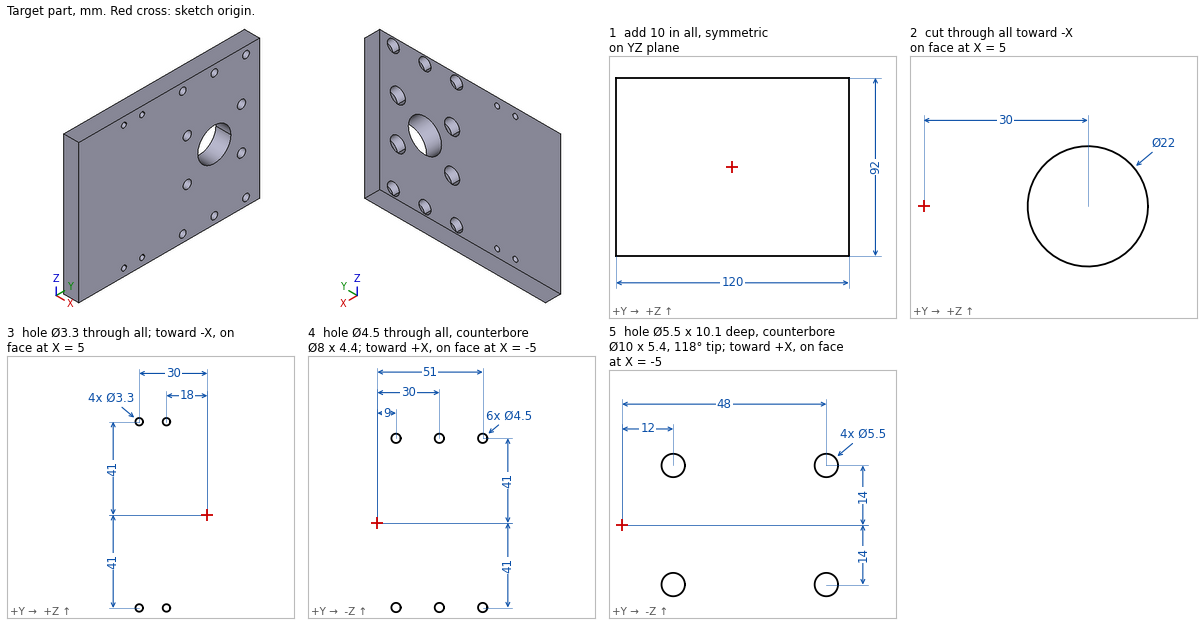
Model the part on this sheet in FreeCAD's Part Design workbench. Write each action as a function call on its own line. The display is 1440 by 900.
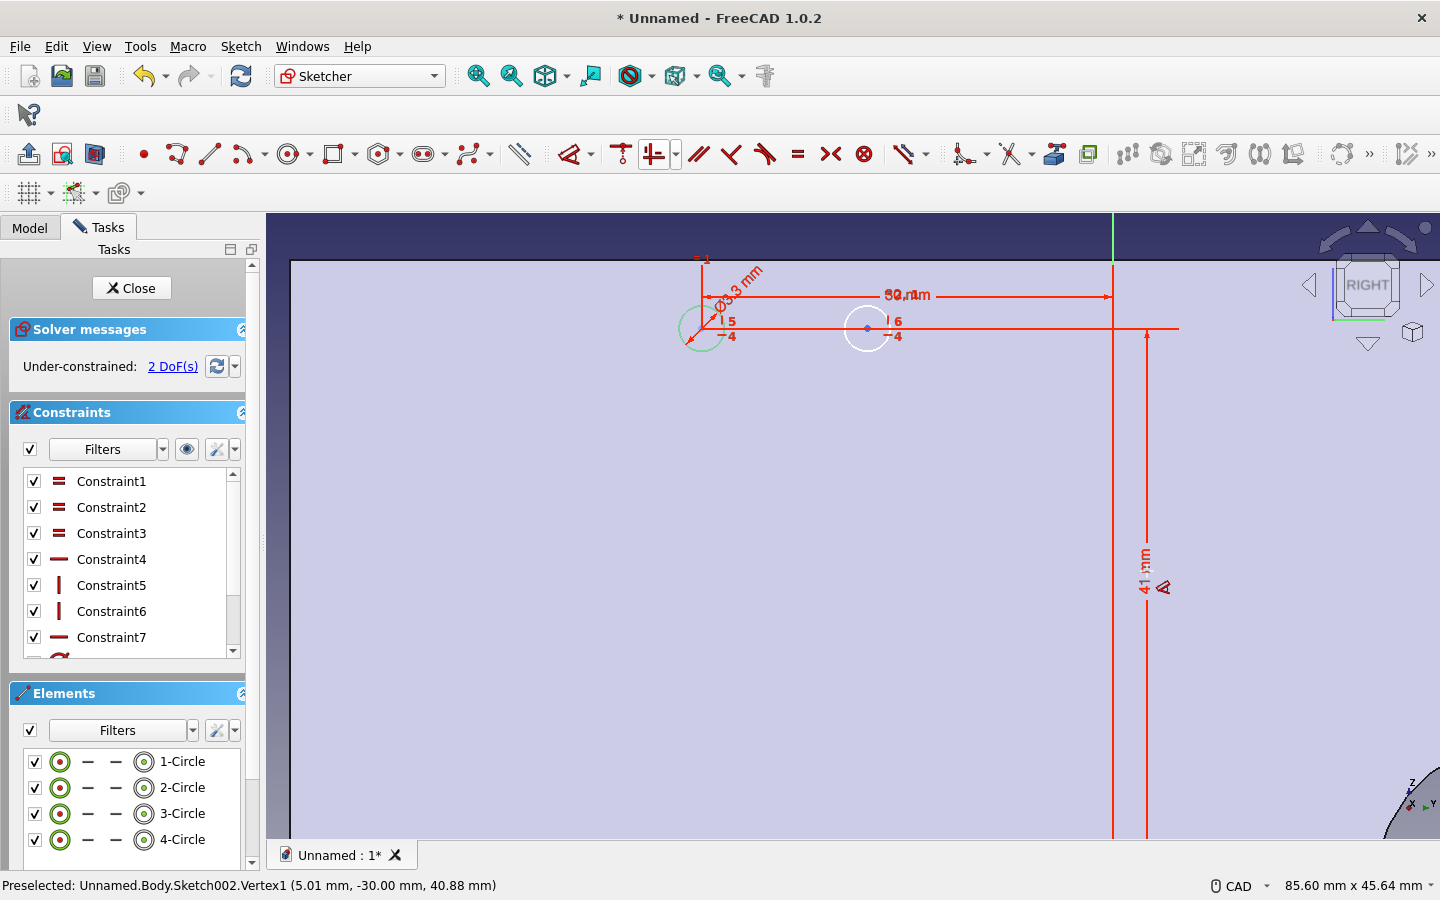
click(867, 329)
click(990, 295)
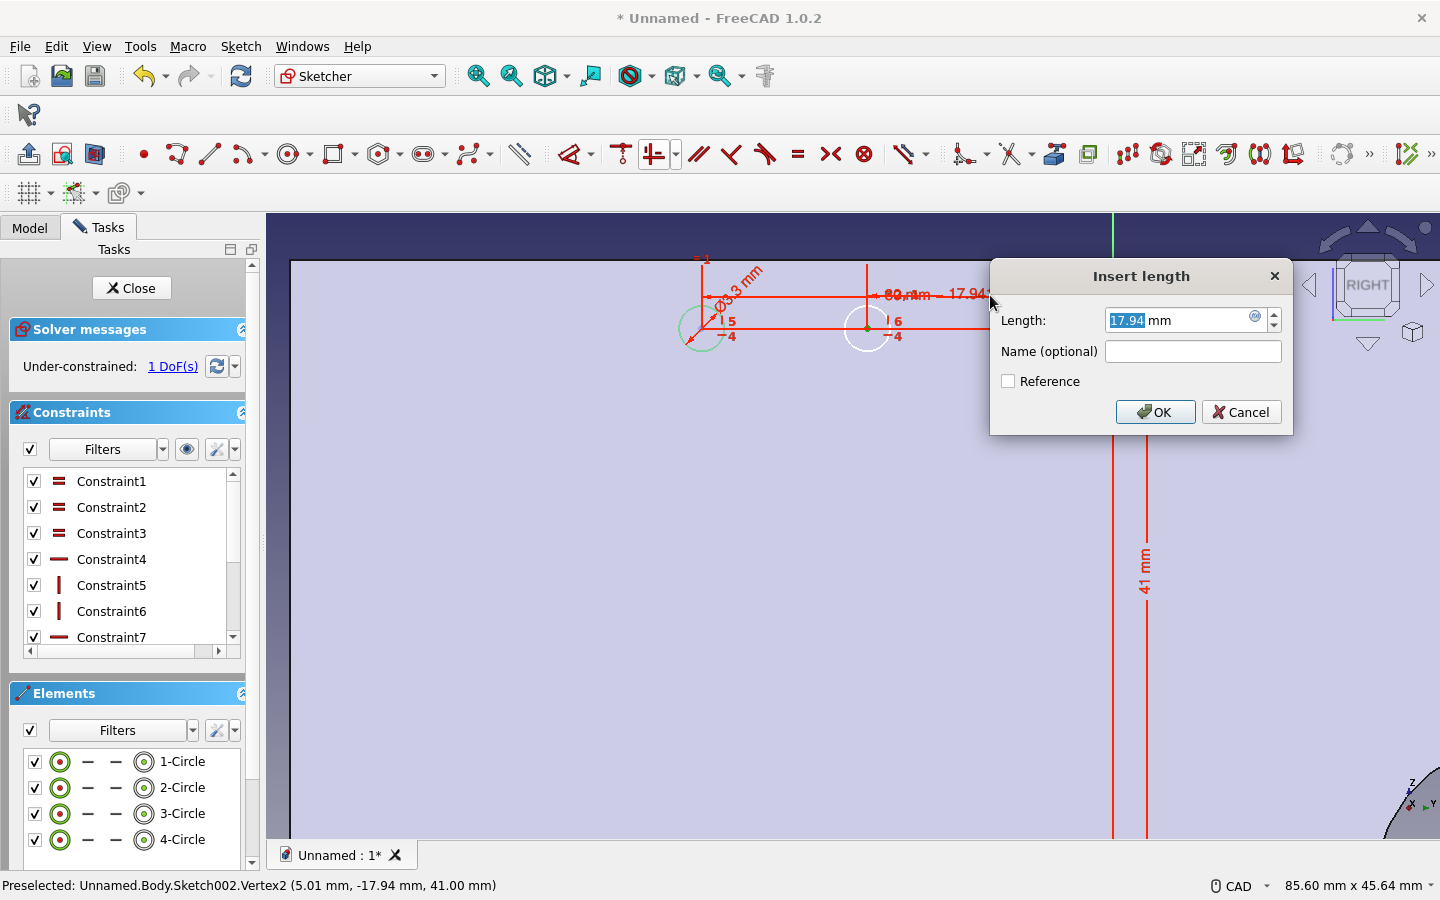
text(18)
key(Return)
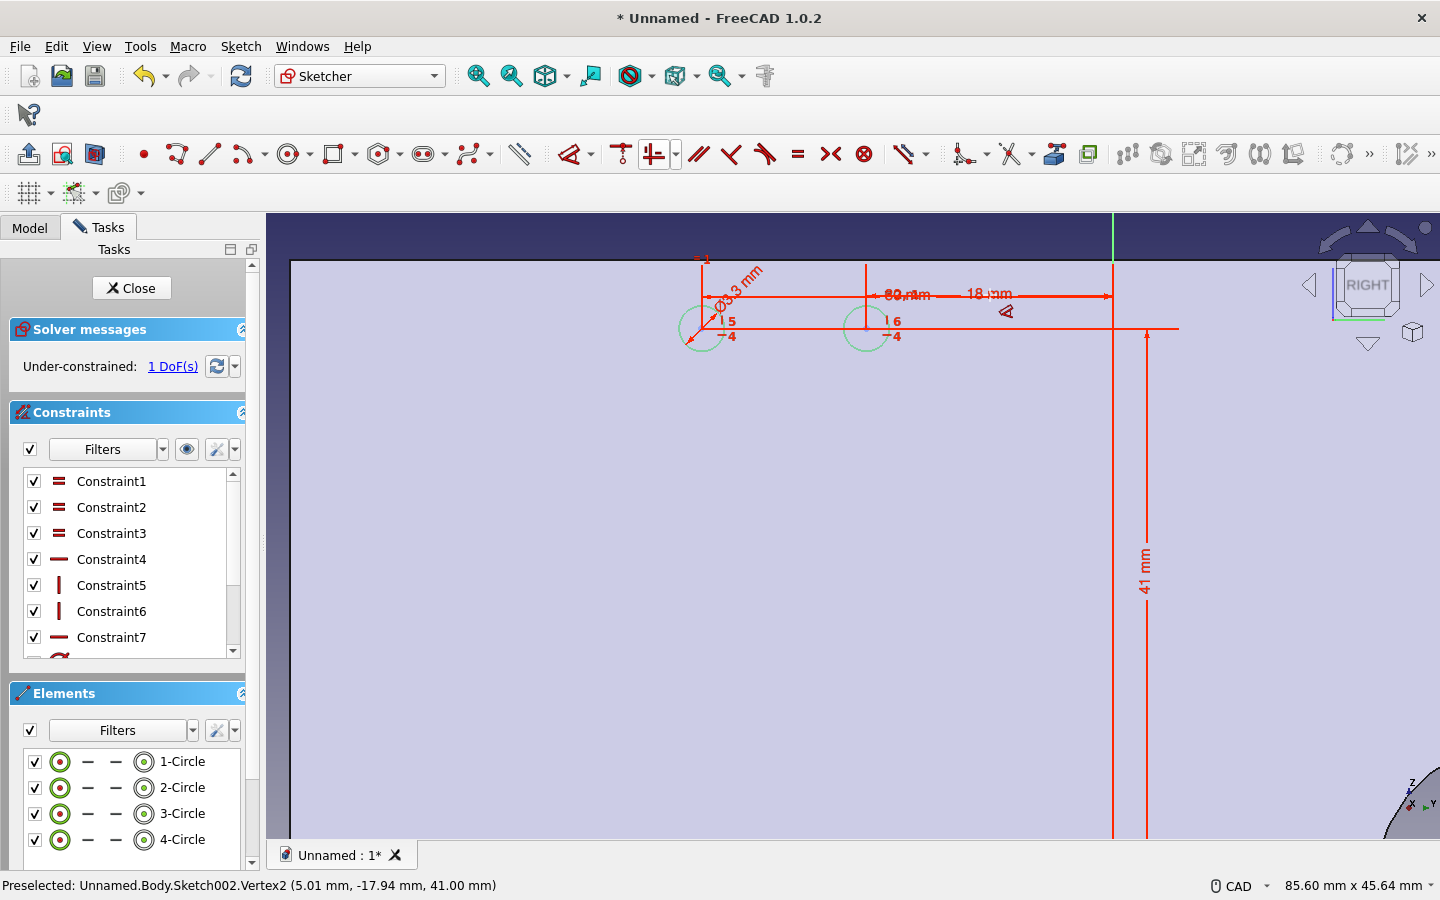
scroll(719, 314, down, 5)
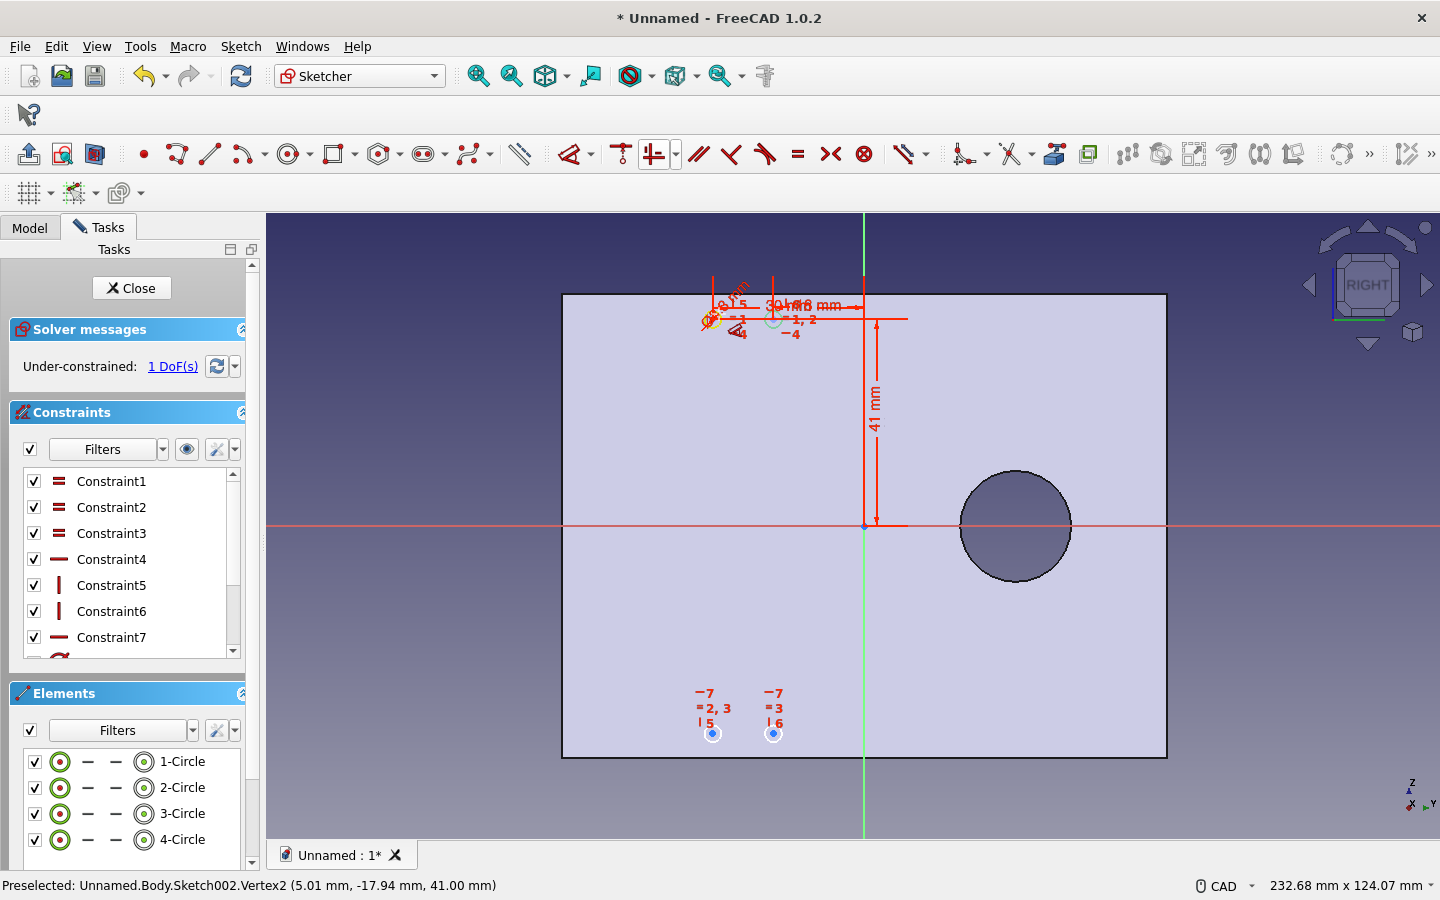
click(713, 734)
click(898, 630)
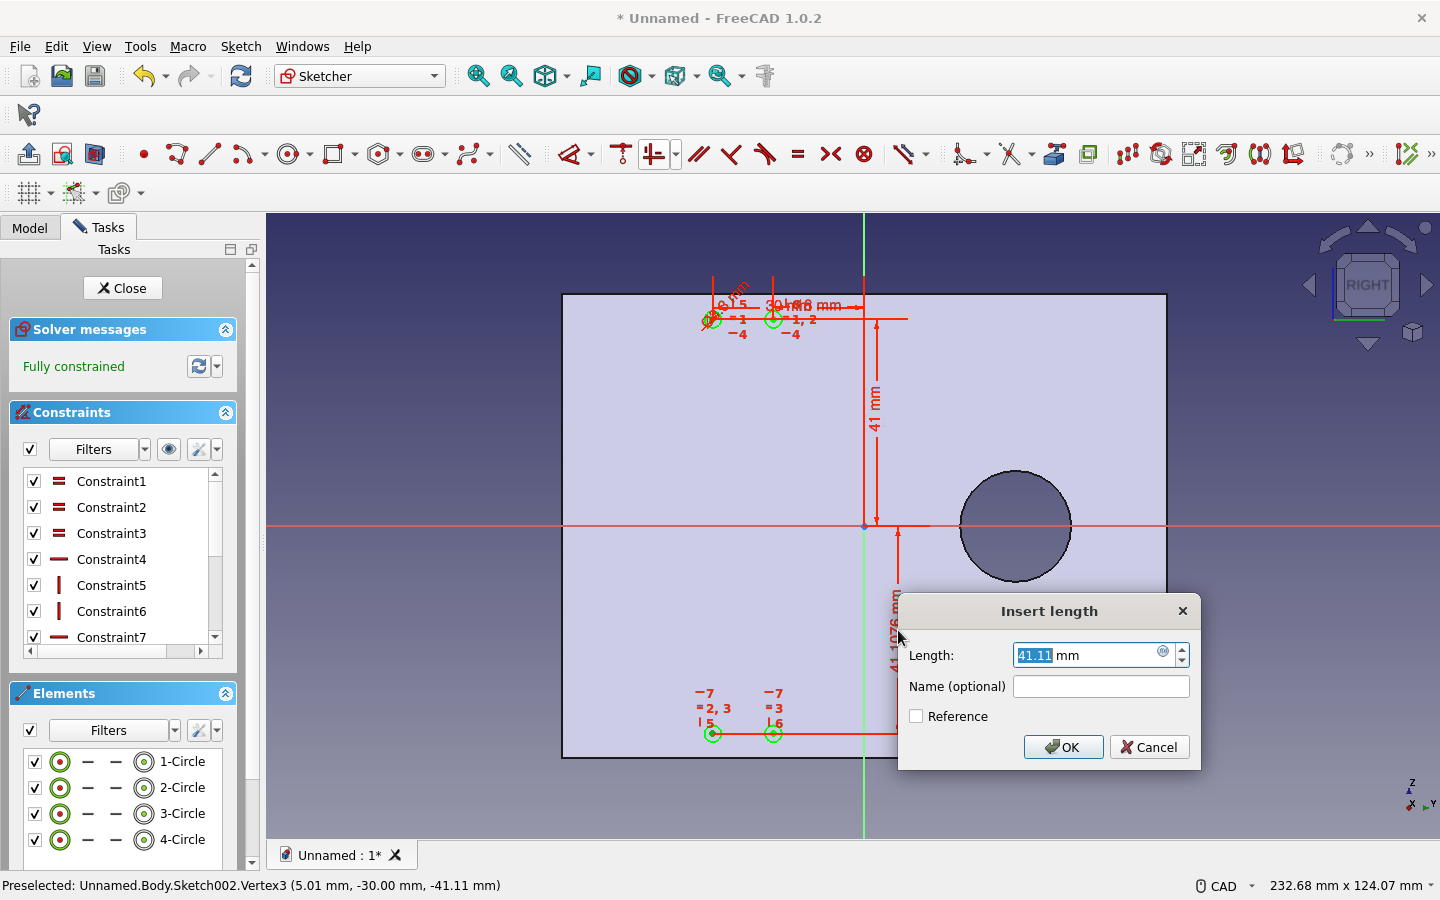
text(41)
key(Return)
key(Escape)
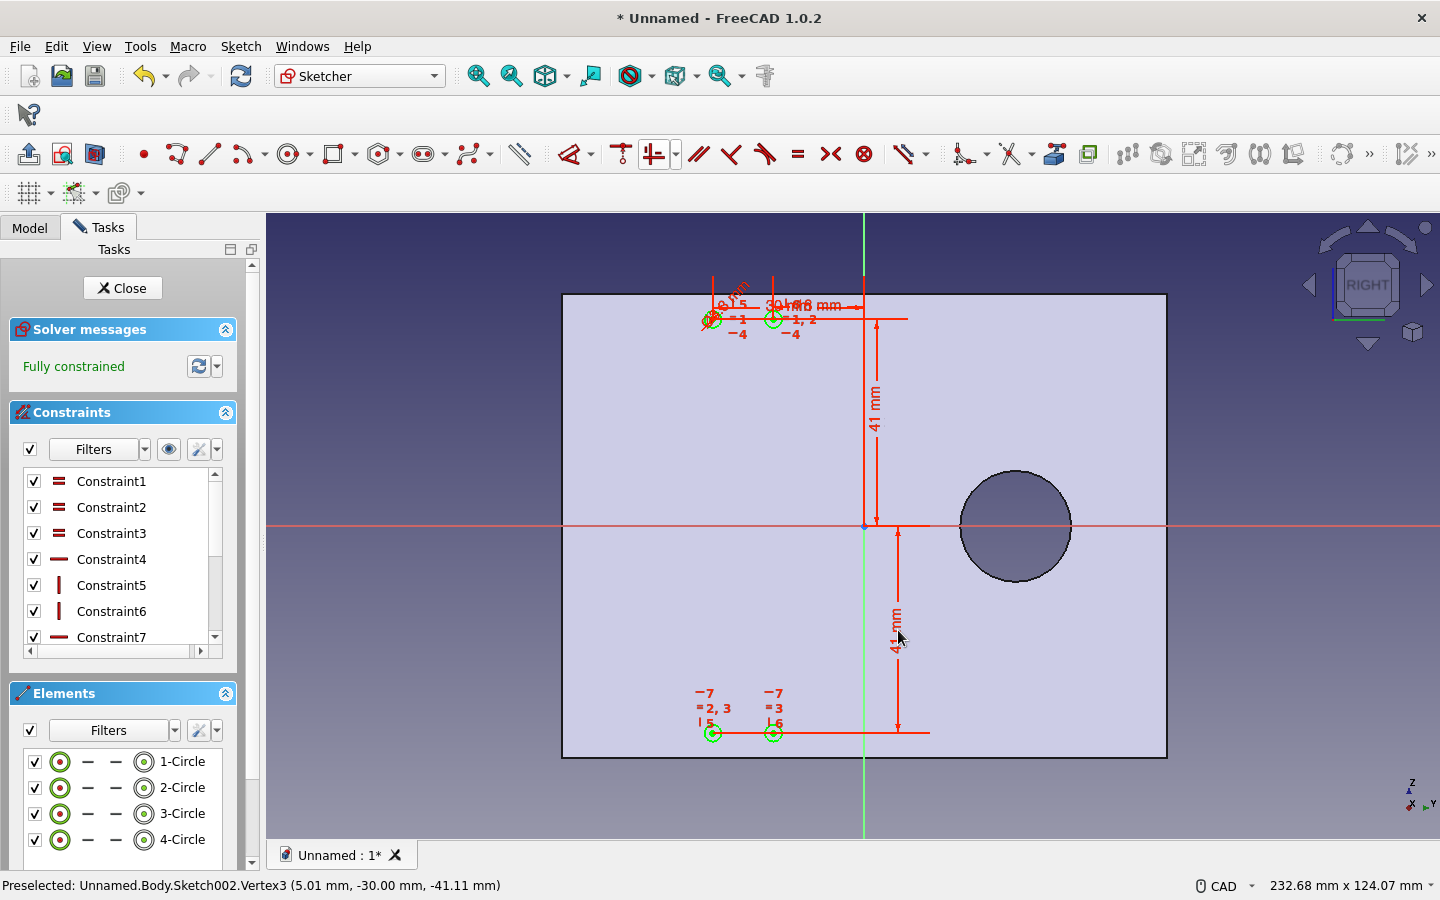
click(123, 288)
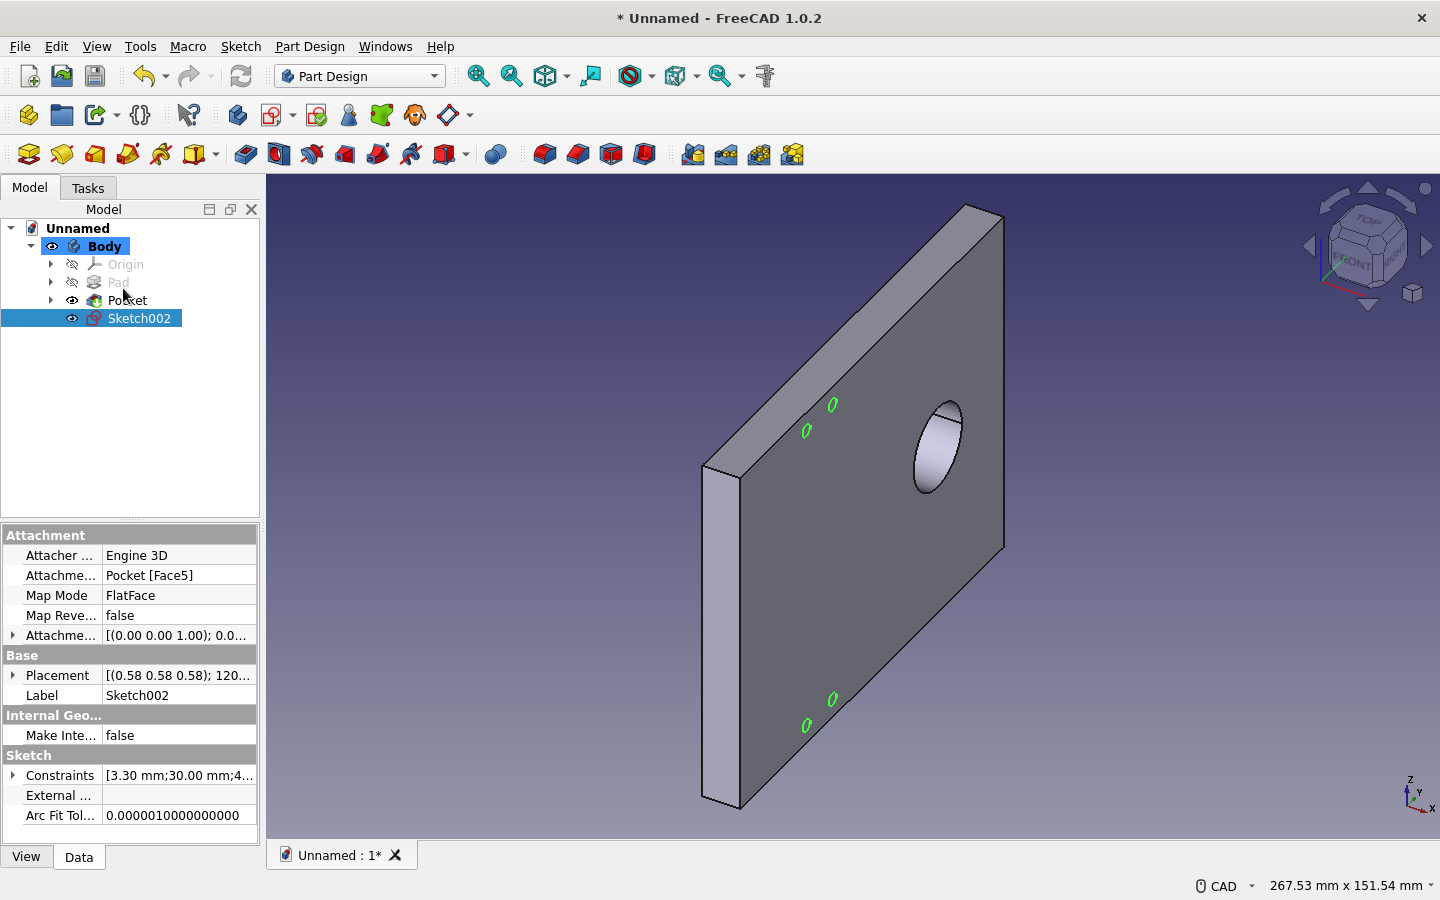
click(279, 154)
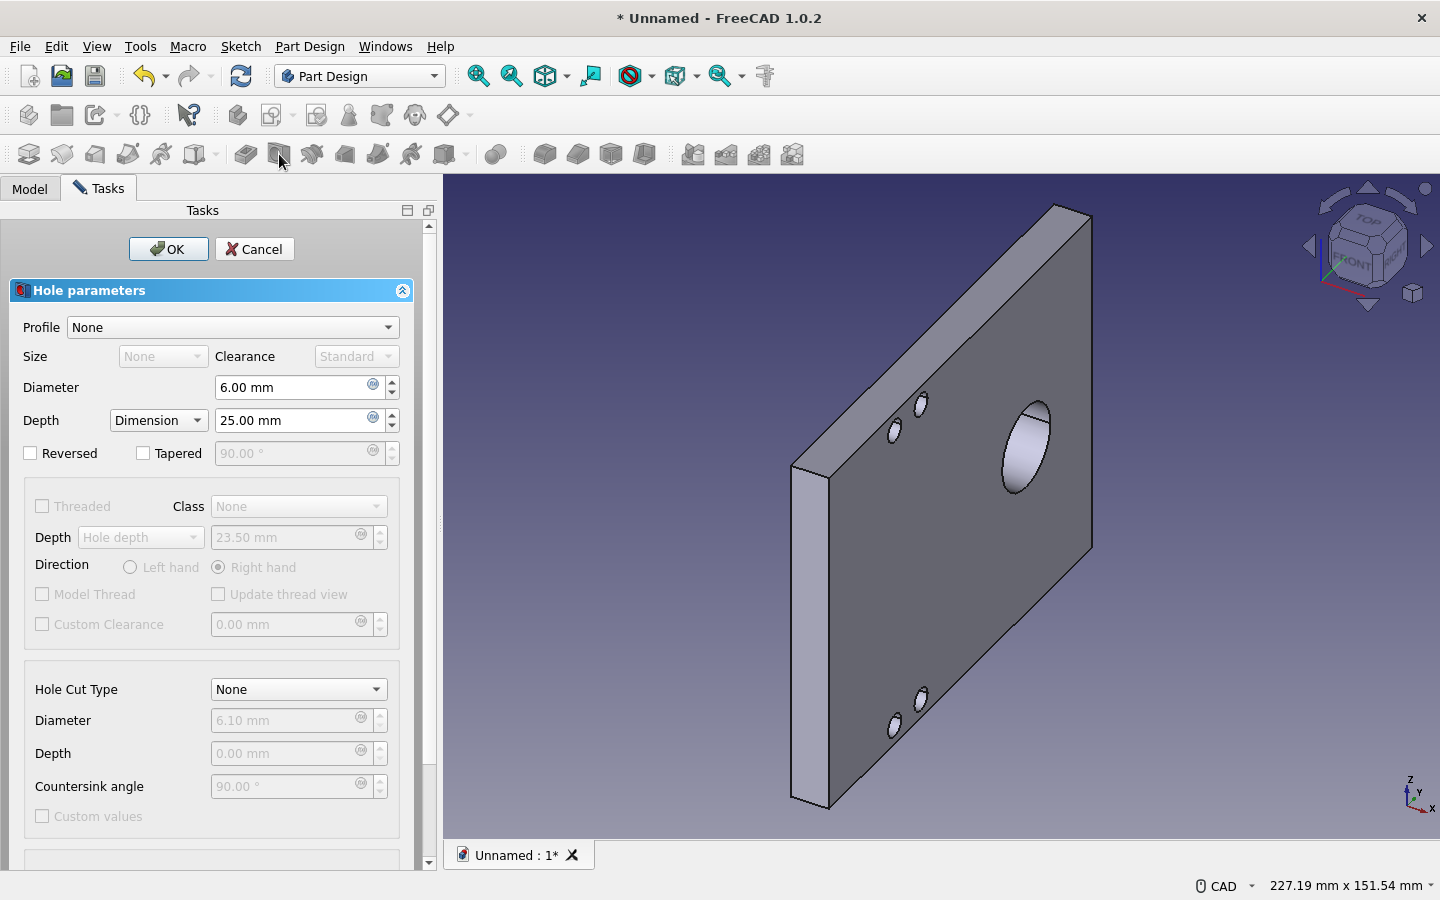
triple_click(300, 388)